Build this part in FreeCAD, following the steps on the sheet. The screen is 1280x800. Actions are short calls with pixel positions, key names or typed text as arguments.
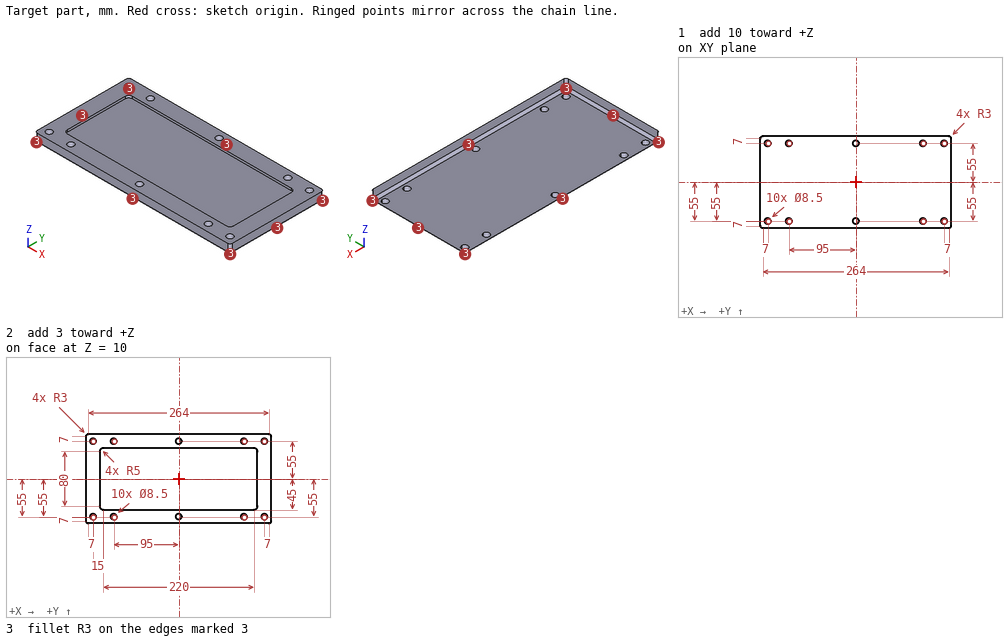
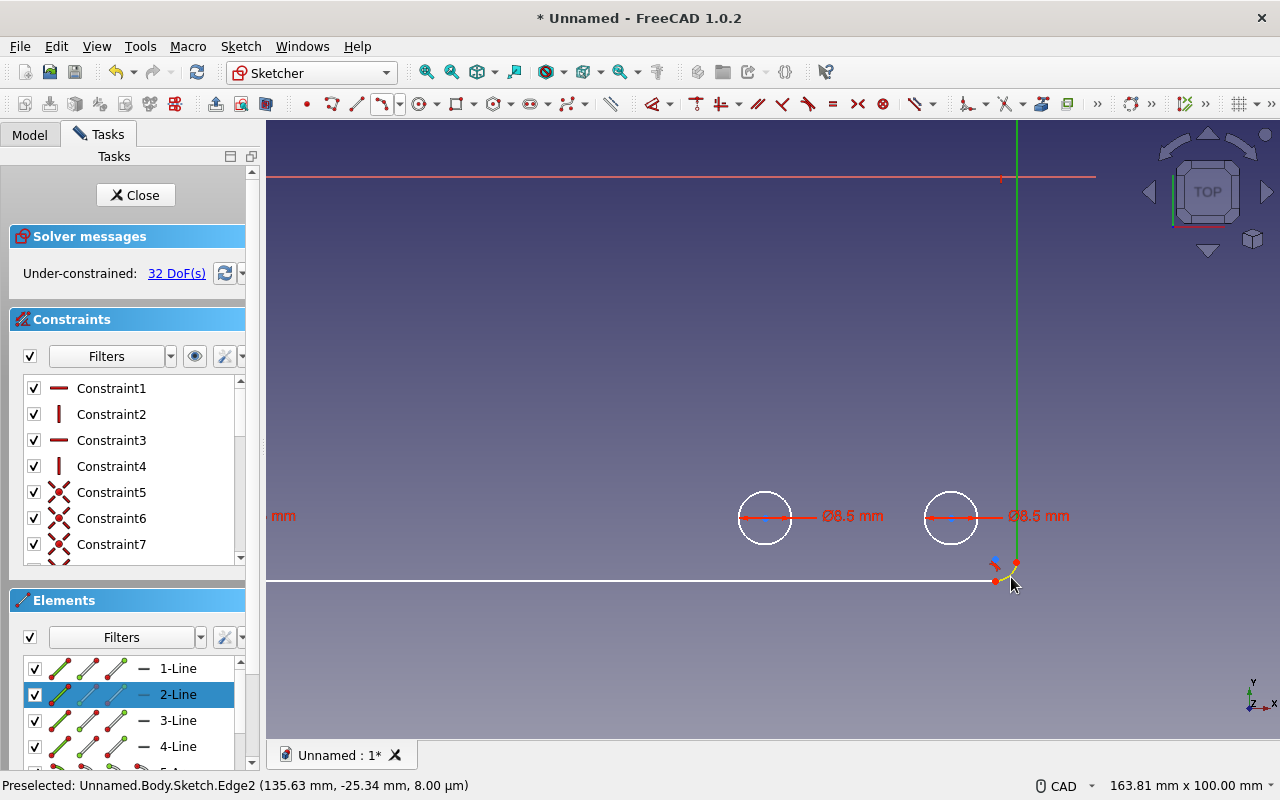
click(1010, 576)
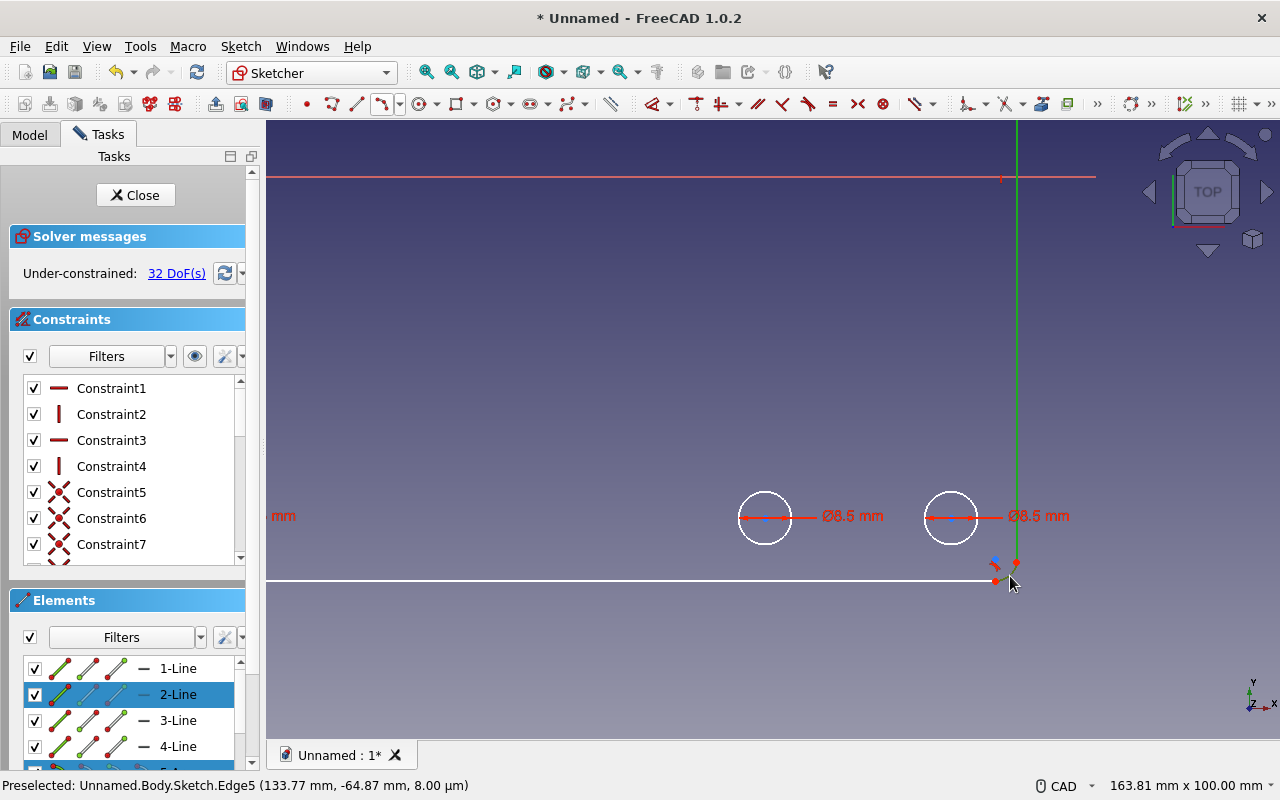
click(808, 104)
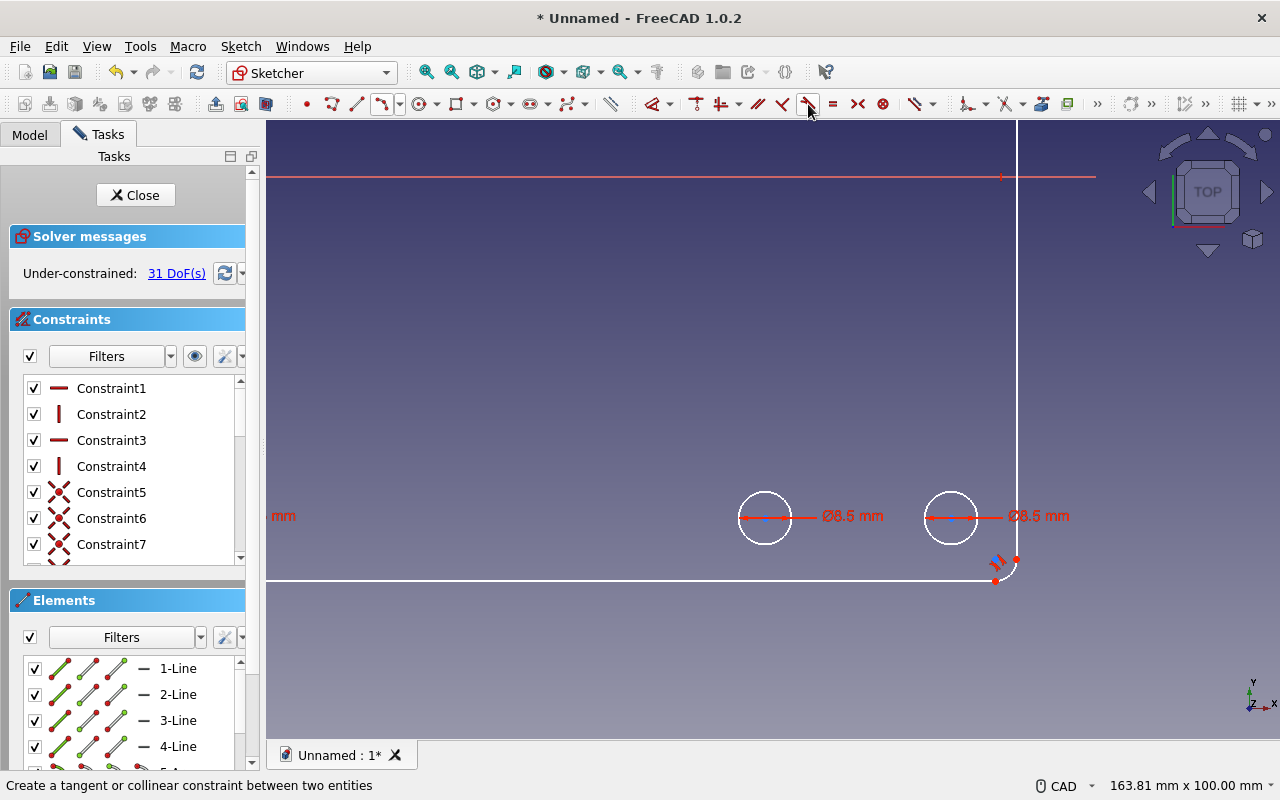
click(1017, 330)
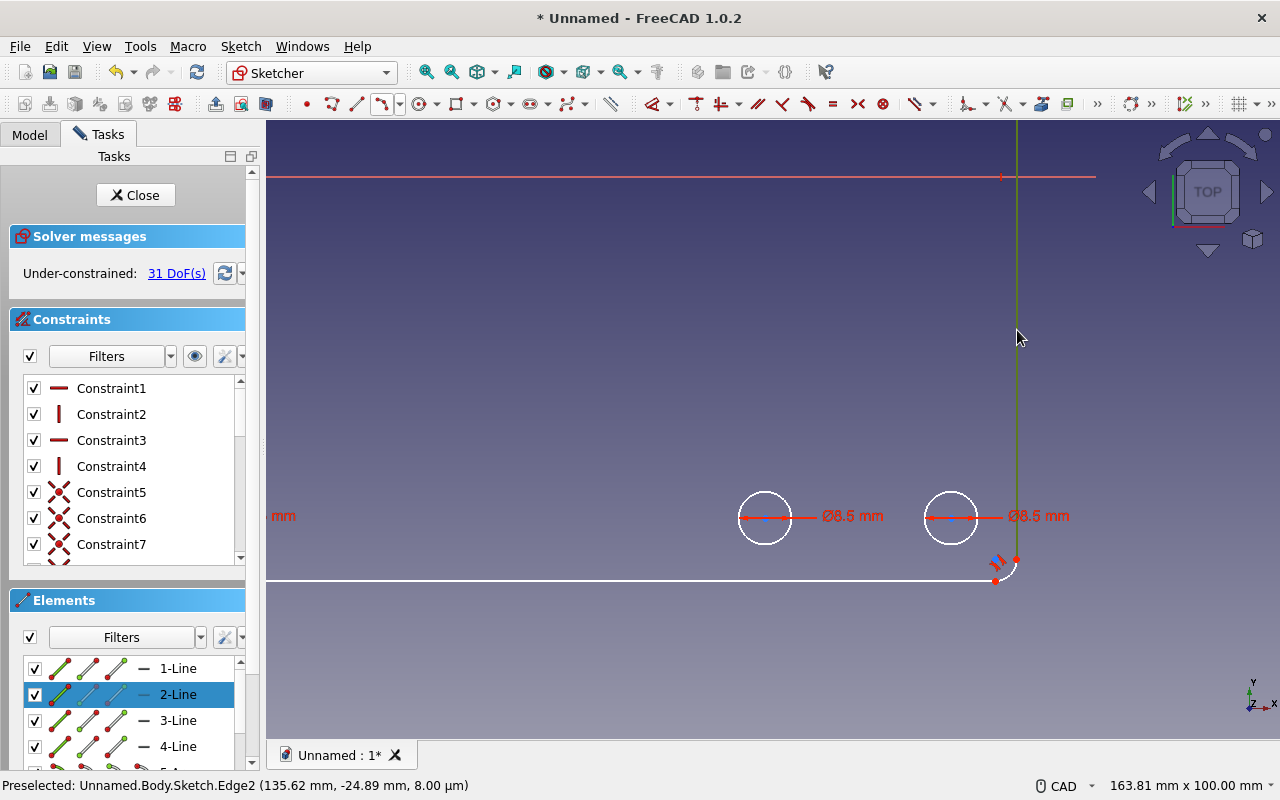
scroll(1011, 576, down, 5)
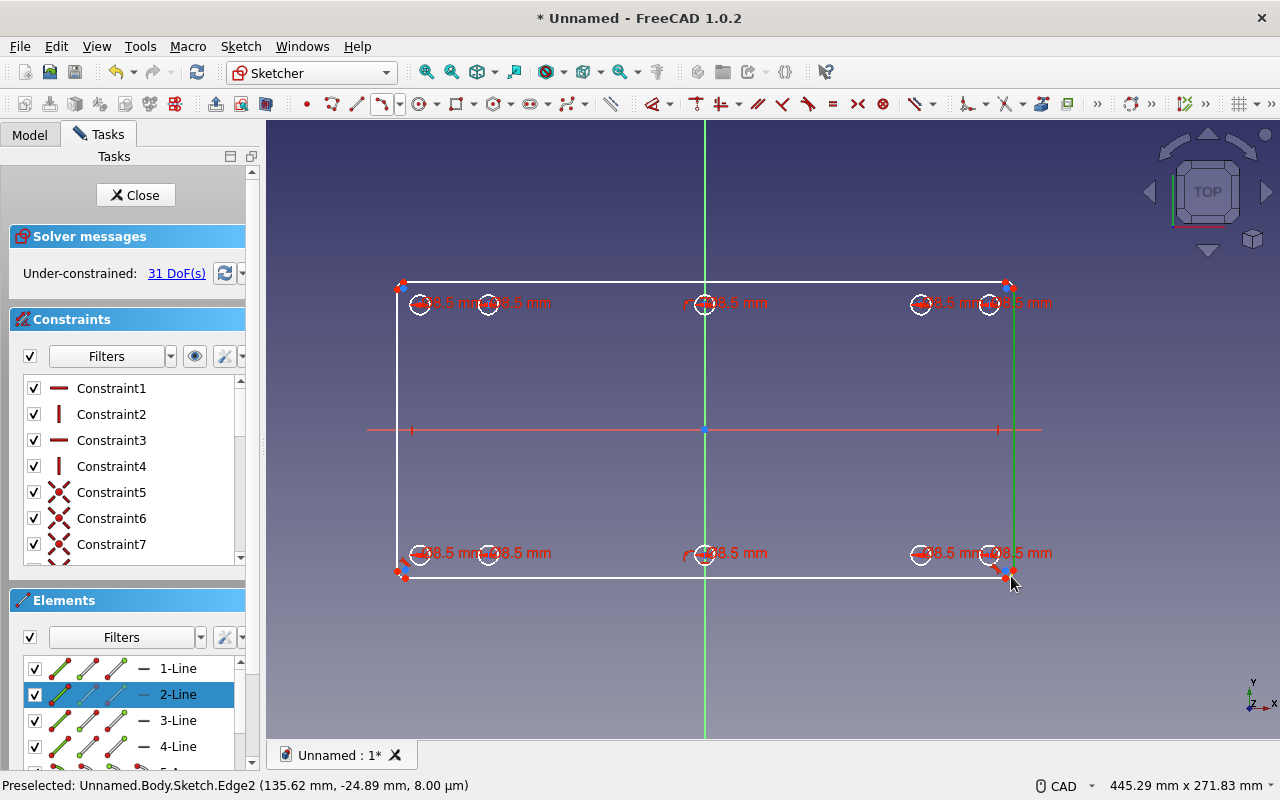
scroll(1013, 285, up, 7)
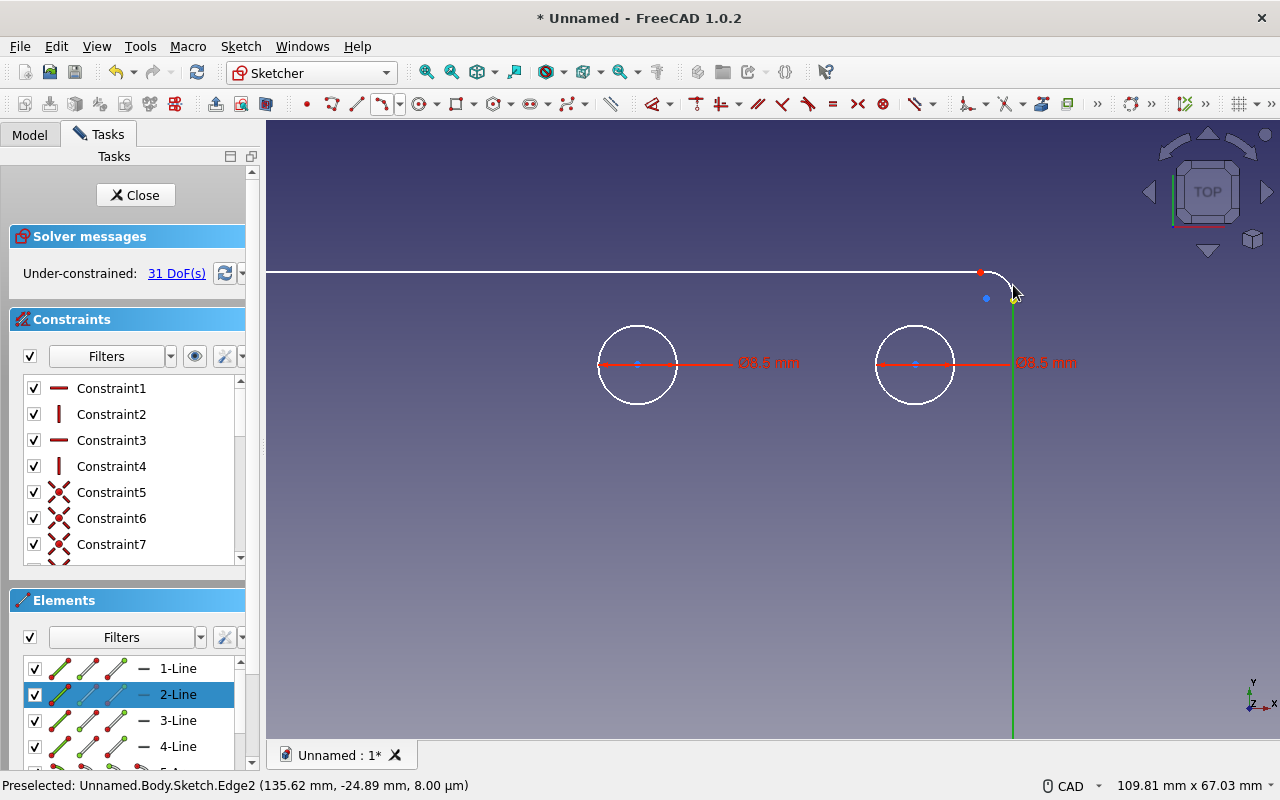
click(1010, 286)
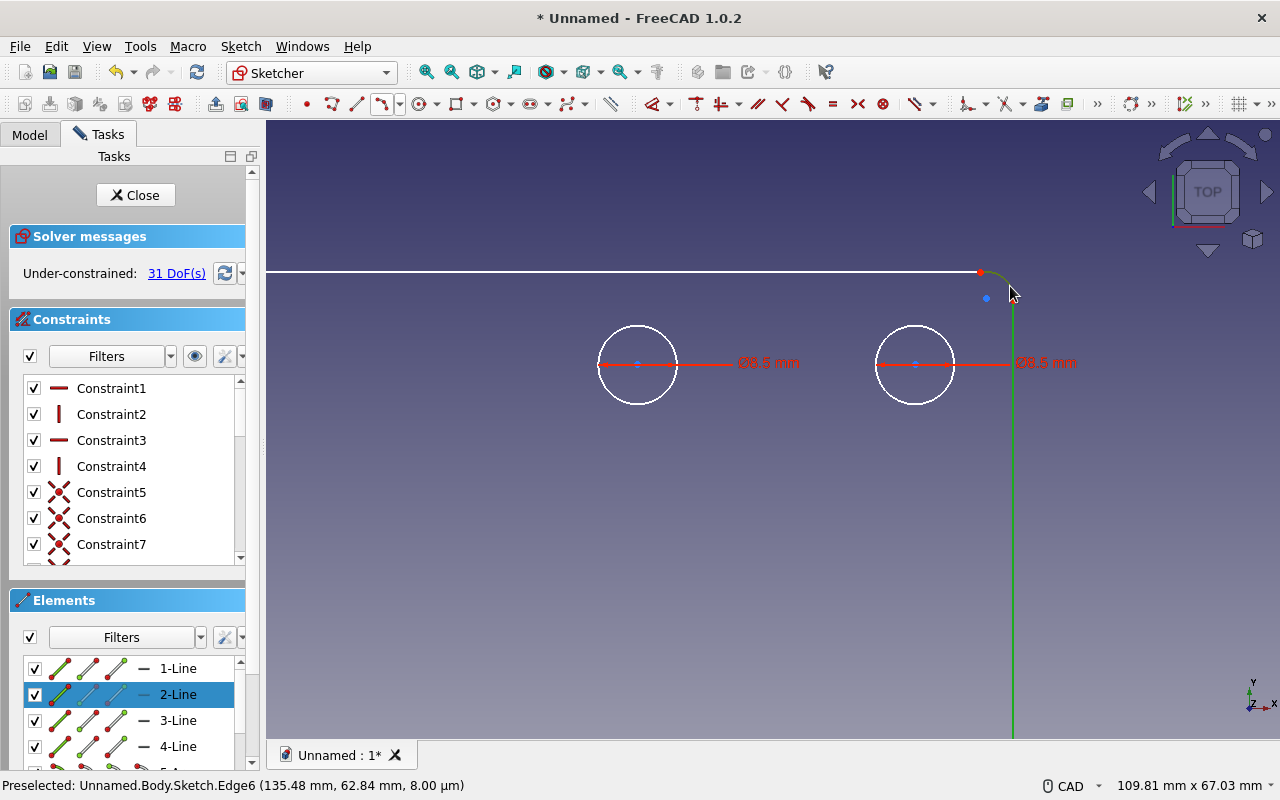
click(808, 104)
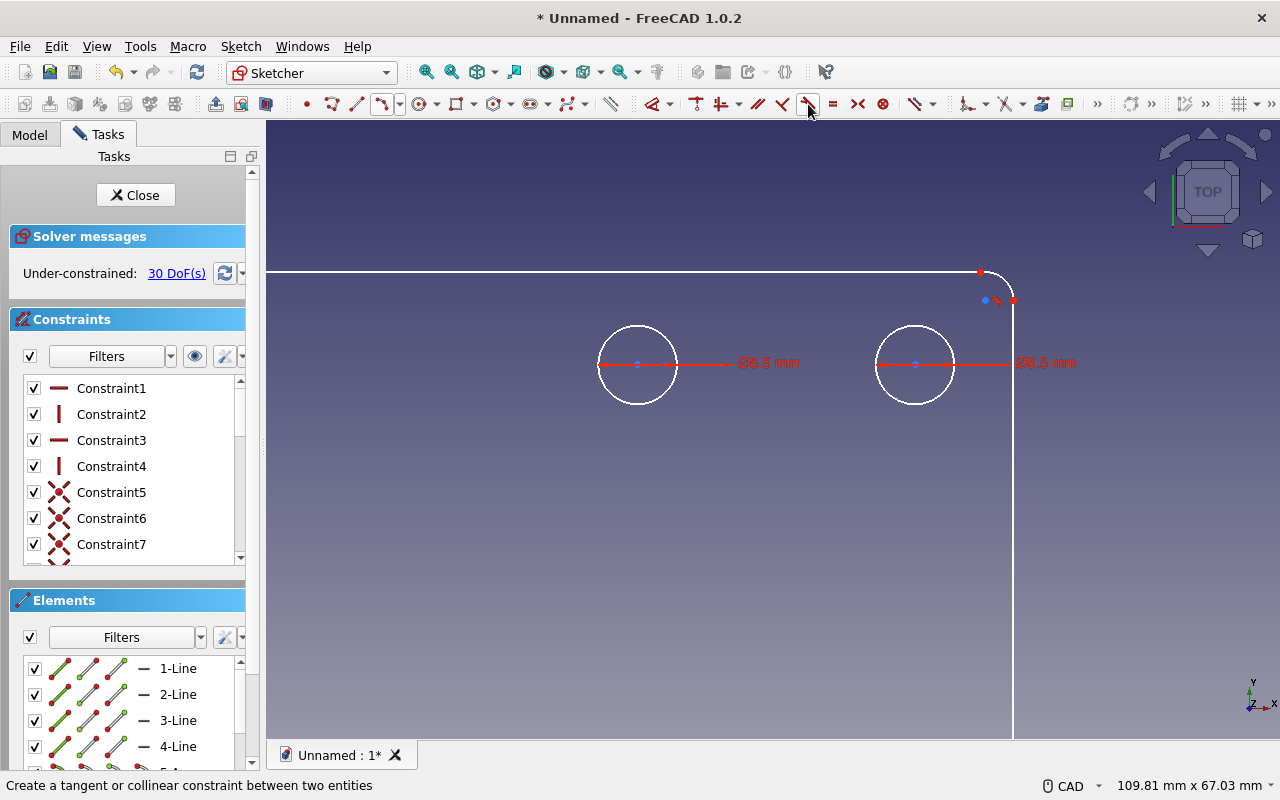
scroll(1013, 285, down, 7)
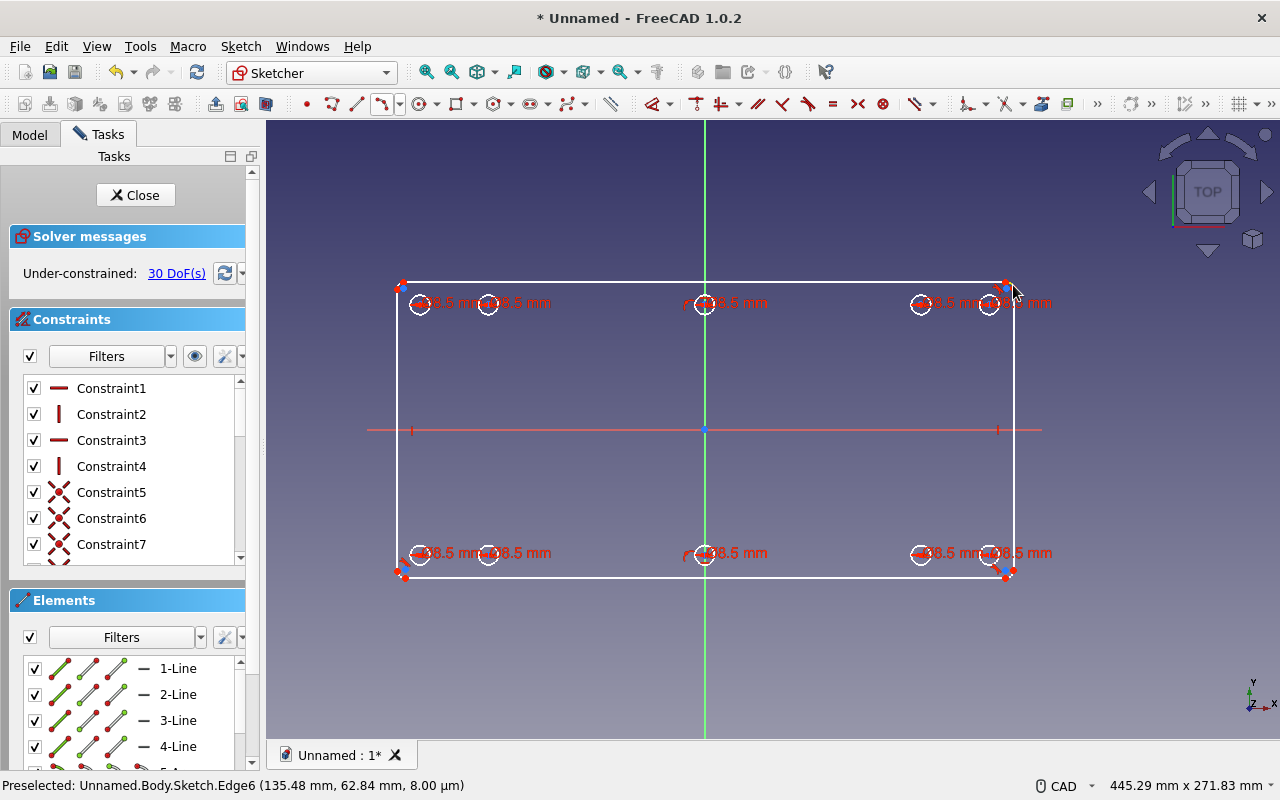
click(885, 282)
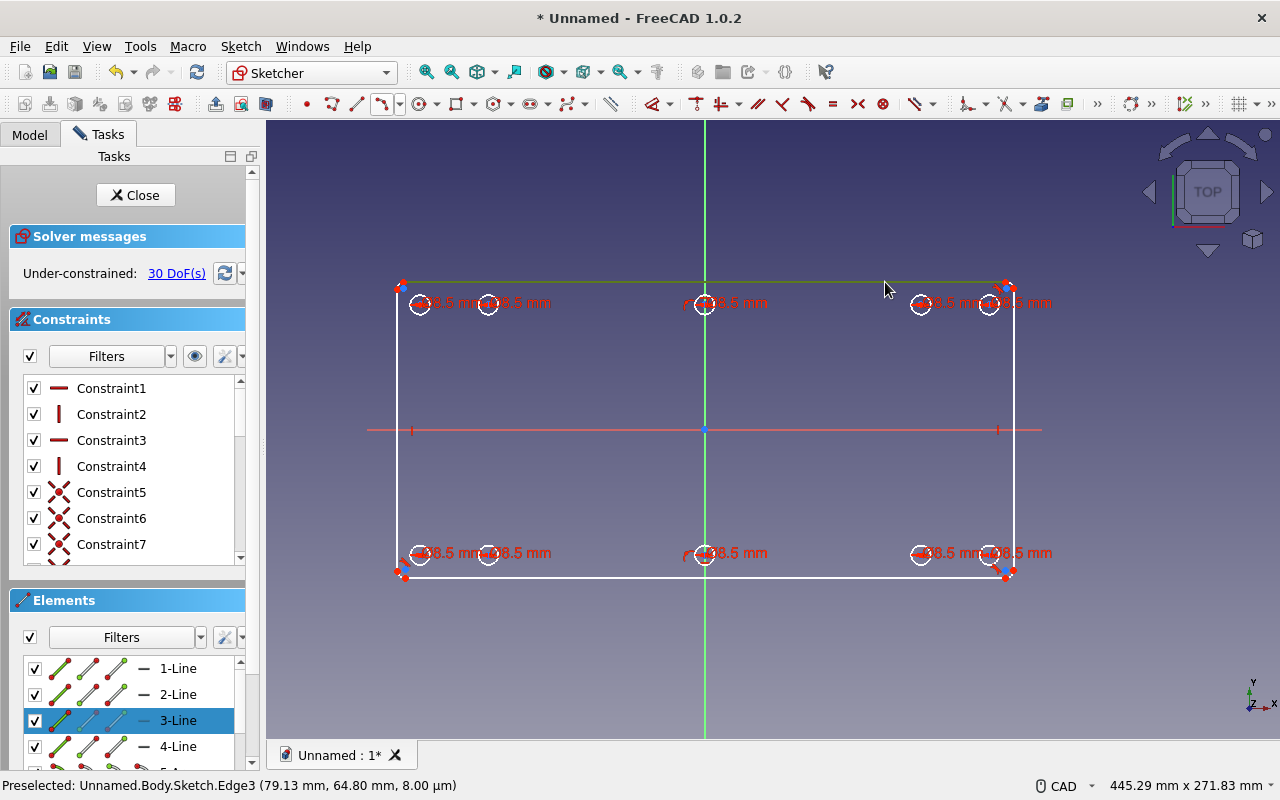
scroll(1011, 284, up, 5)